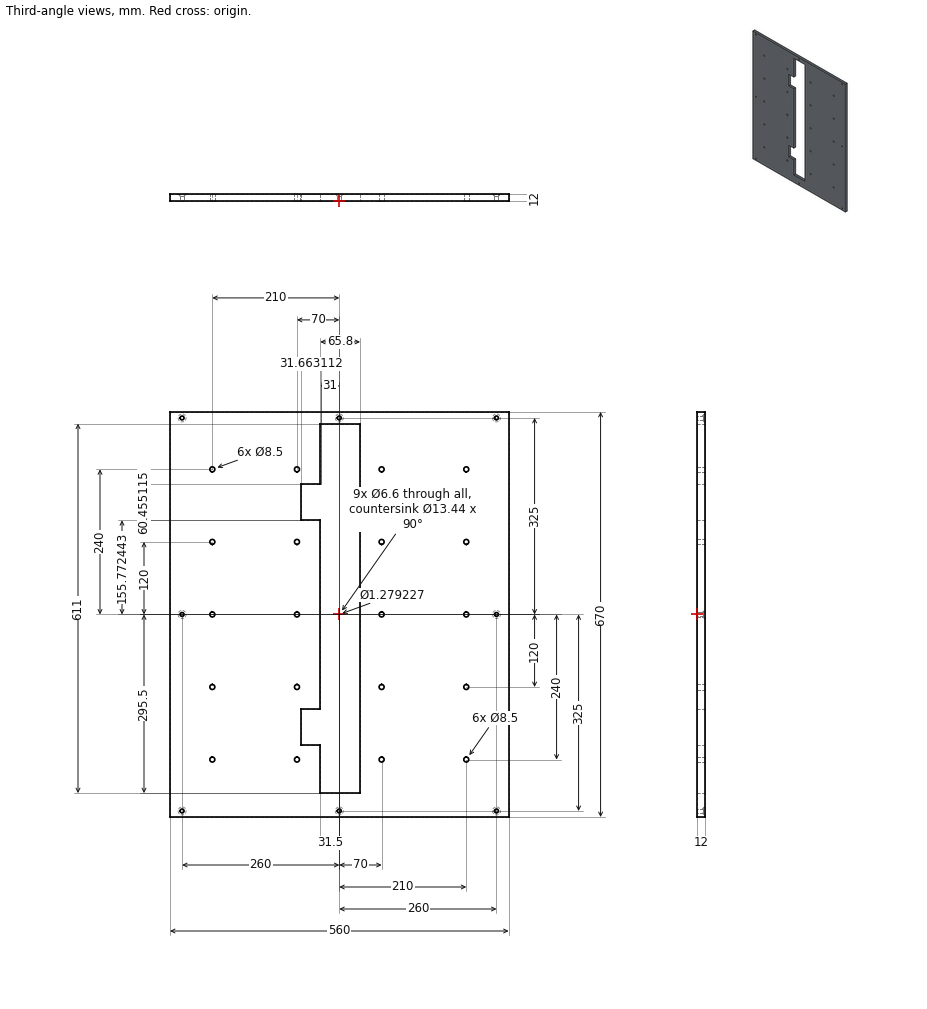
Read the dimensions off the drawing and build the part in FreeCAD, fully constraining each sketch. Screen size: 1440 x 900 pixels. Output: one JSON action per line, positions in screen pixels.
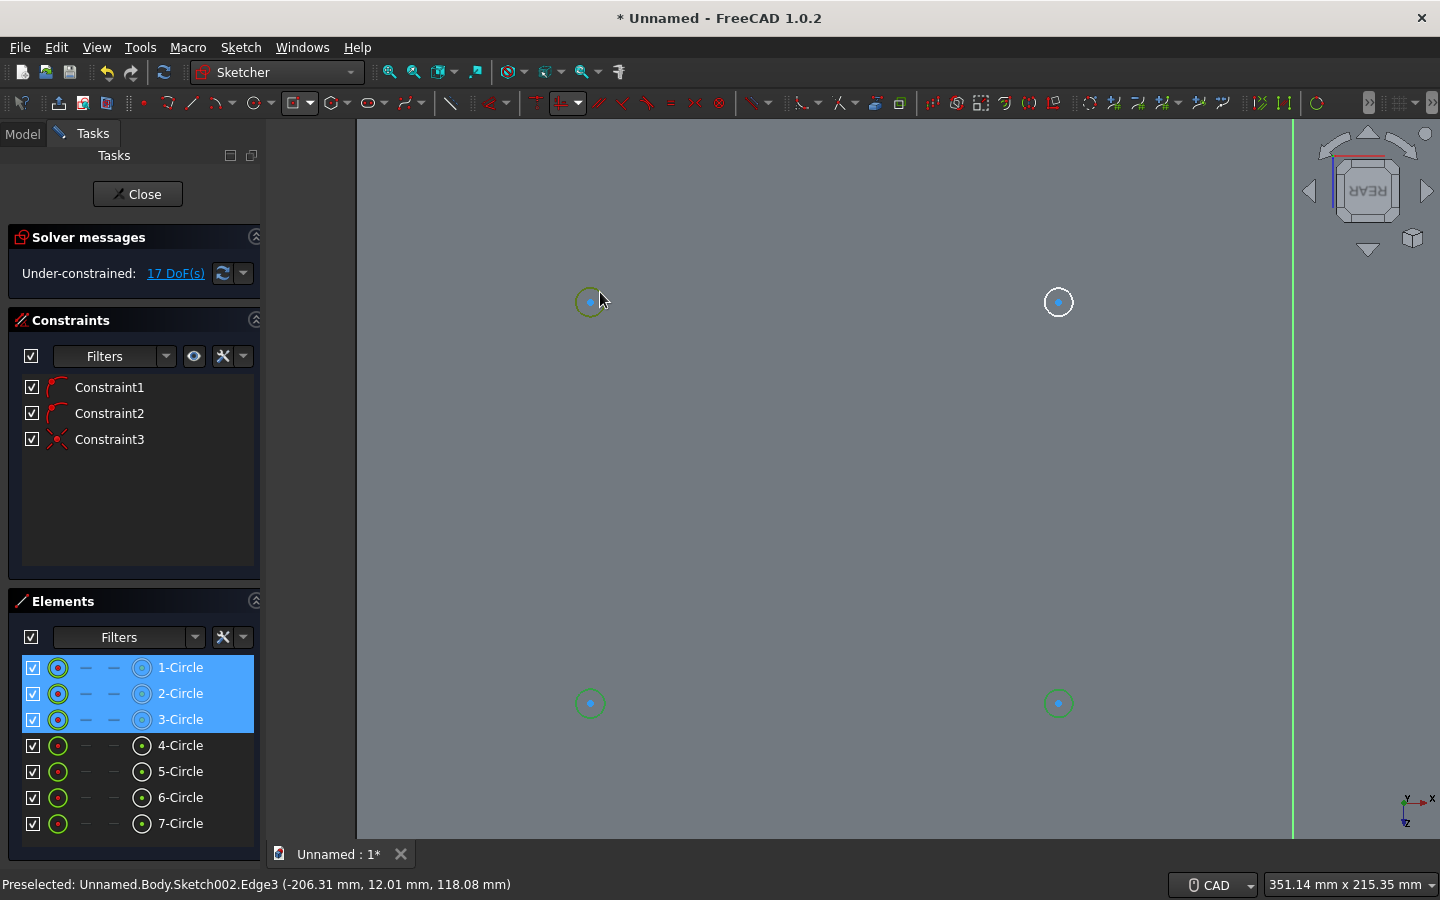
{"action": "left_click", "coordinate": [1069, 292]}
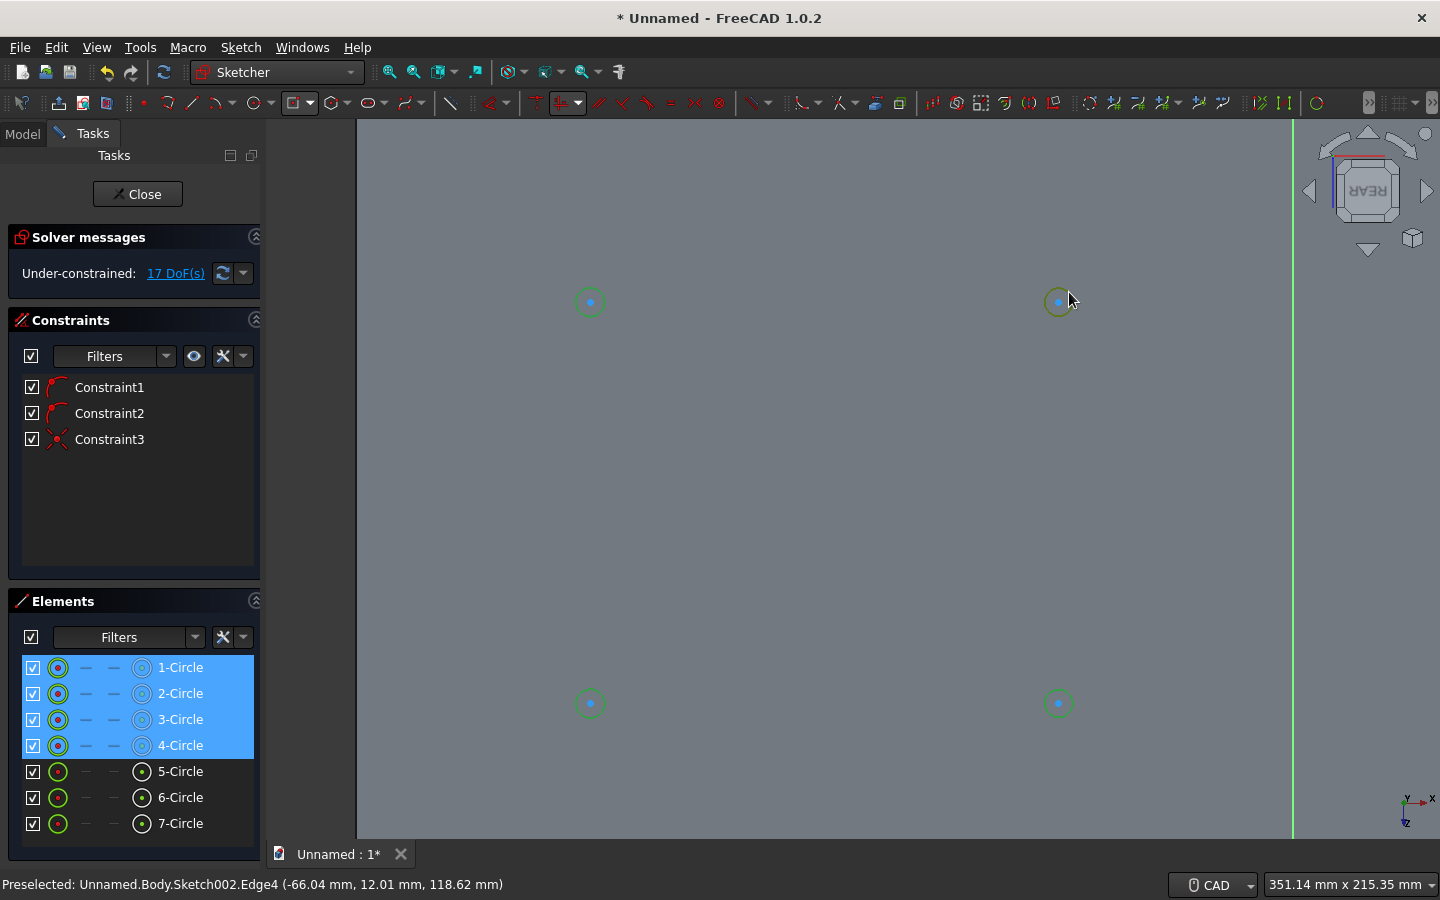
{"action": "scroll", "coordinate": [601, 695], "scroll_direction": "down", "scroll_amount": 3}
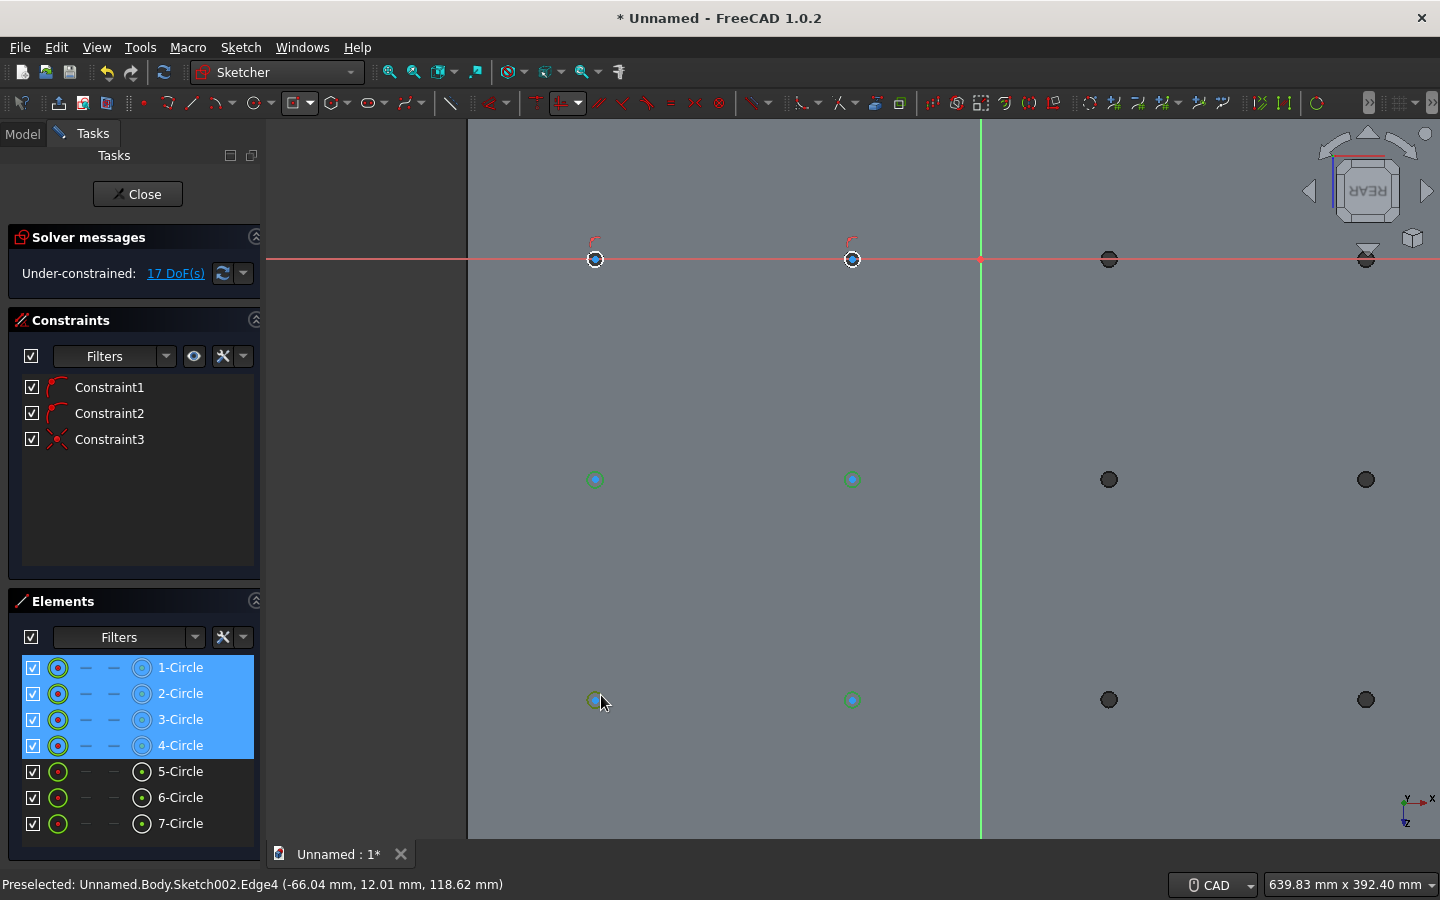
{"action": "scroll", "coordinate": [858, 254], "scroll_direction": "up", "scroll_amount": 5}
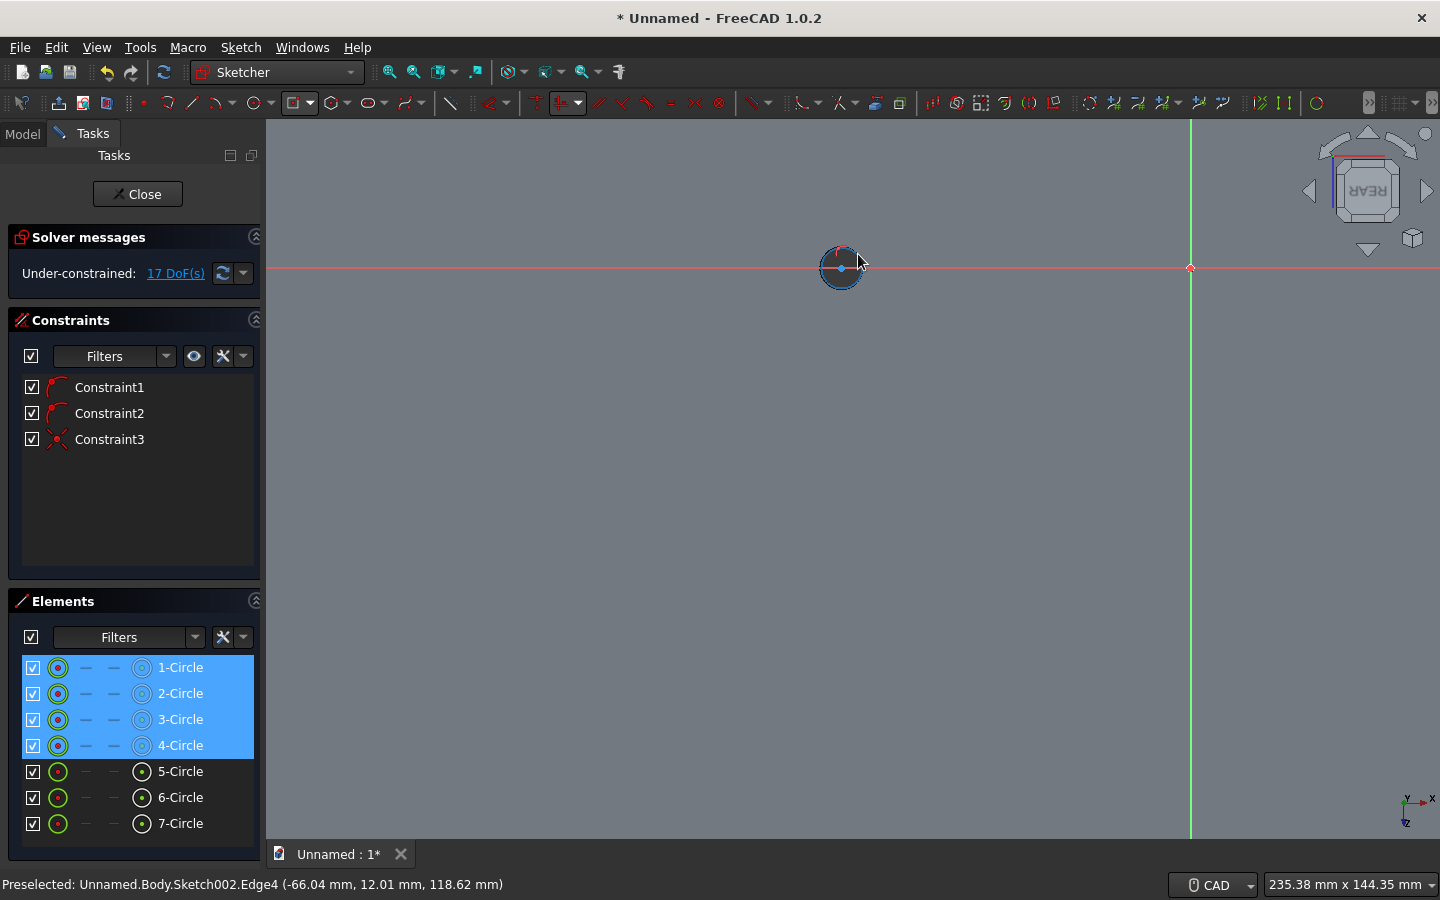
{"action": "left_click", "coordinate": [856, 254]}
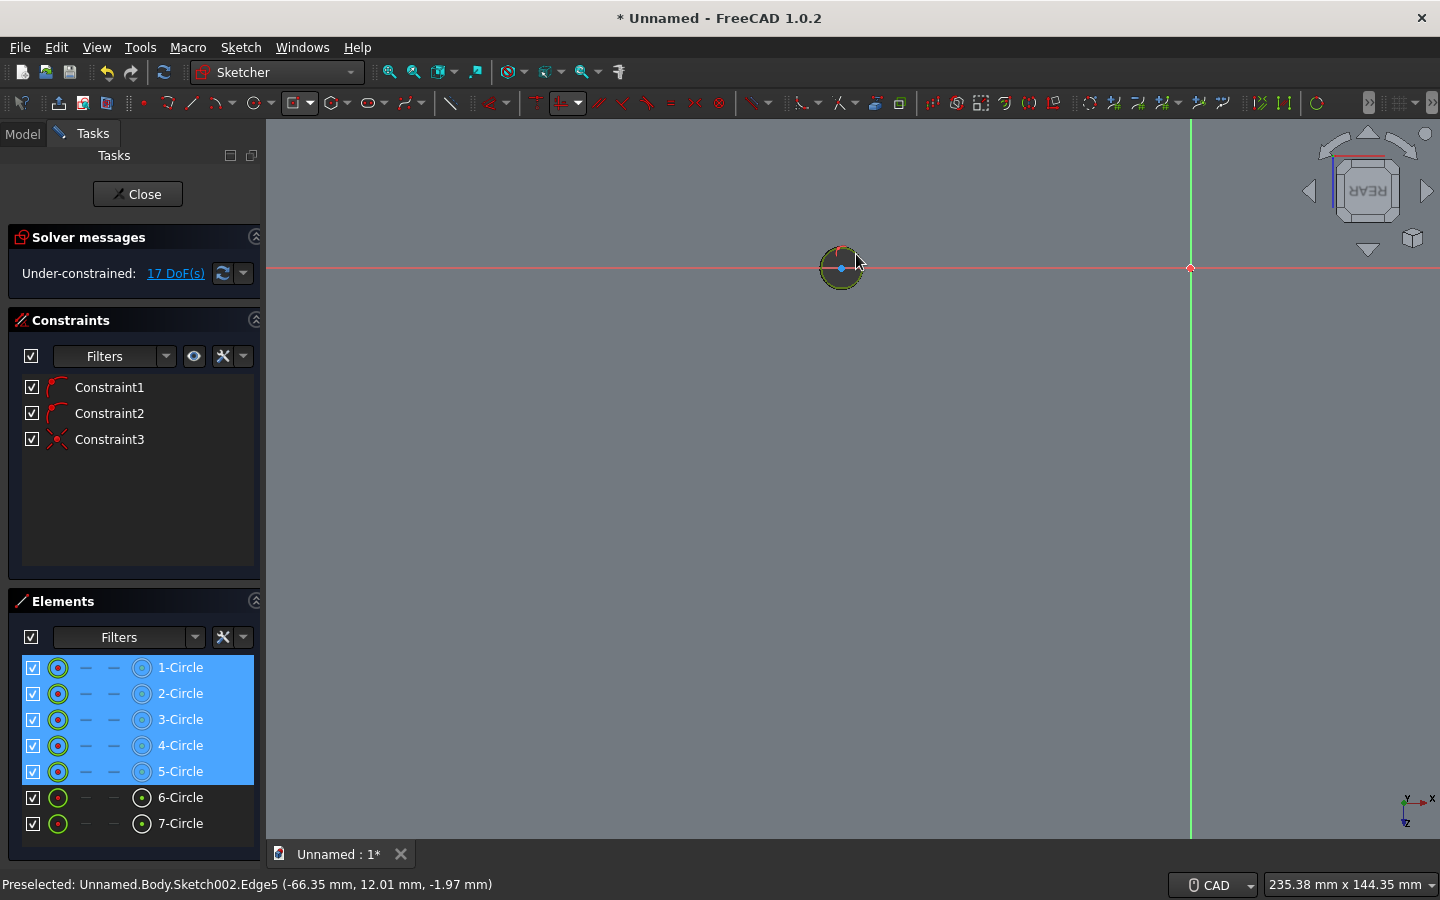
{"action": "scroll", "coordinate": [858, 253], "scroll_direction": "down", "scroll_amount": 5}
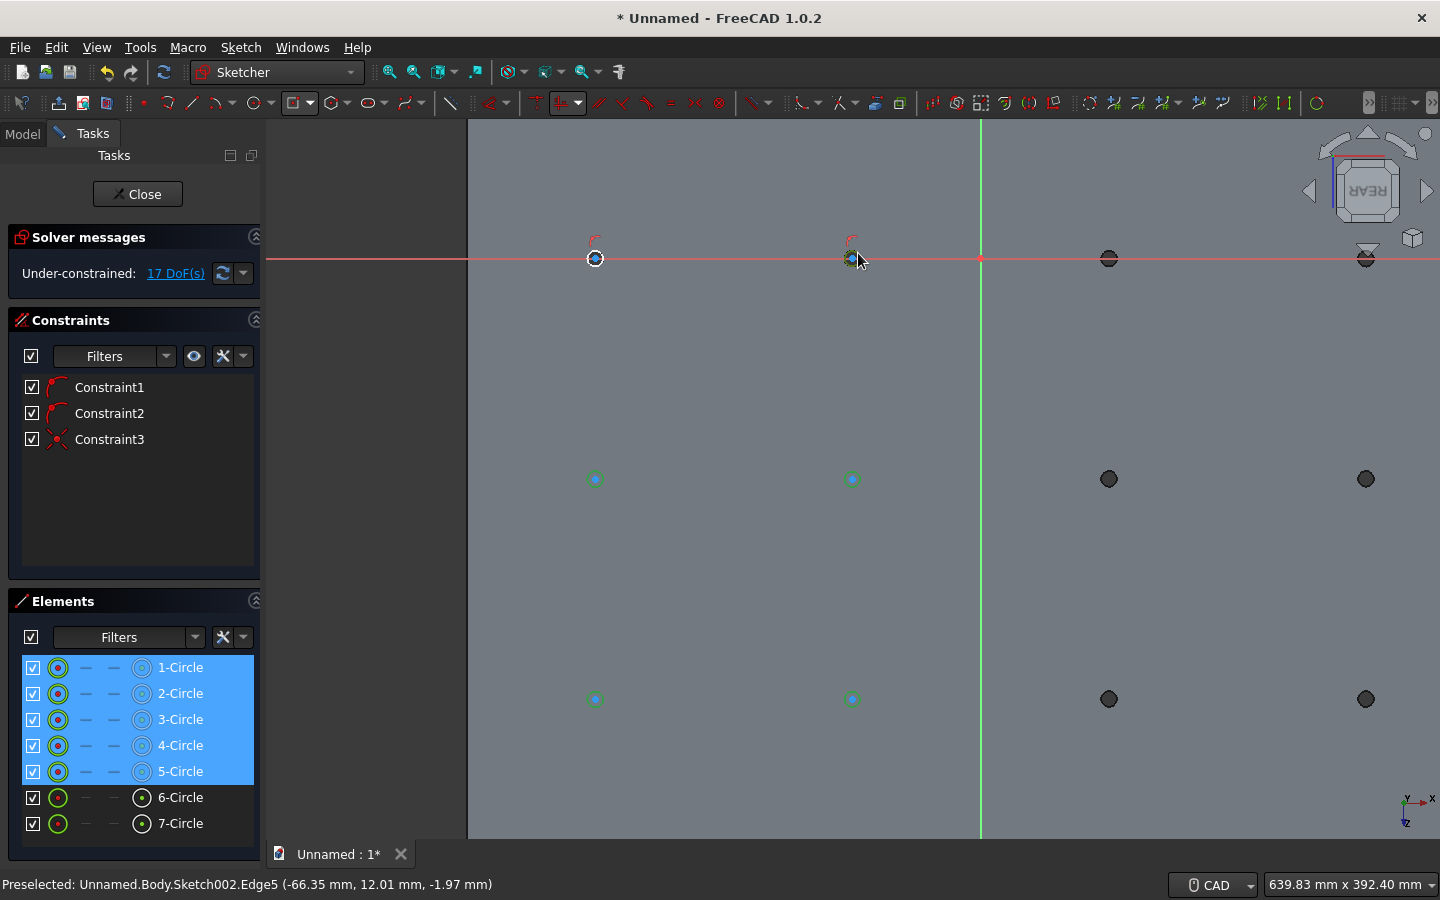
{"action": "scroll", "coordinate": [601, 253], "scroll_direction": "up", "scroll_amount": 5}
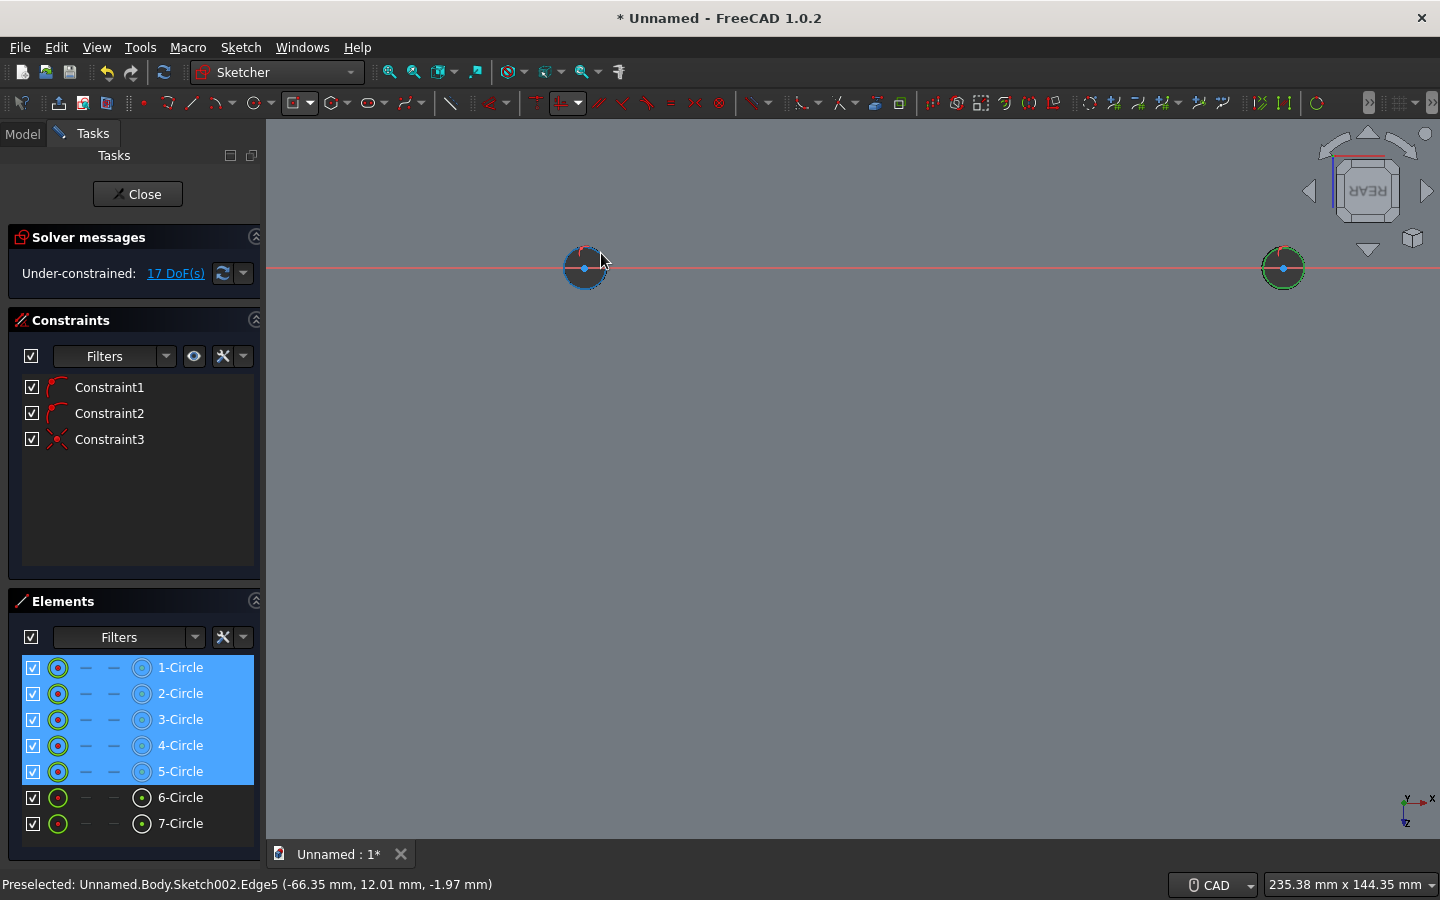
{"action": "left_click", "coordinate": [600, 253]}